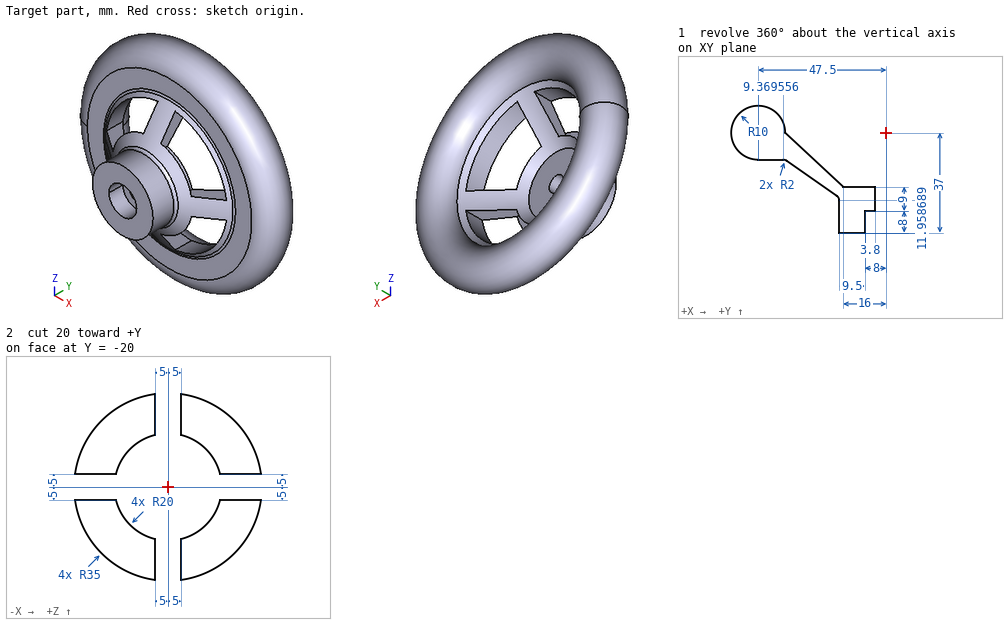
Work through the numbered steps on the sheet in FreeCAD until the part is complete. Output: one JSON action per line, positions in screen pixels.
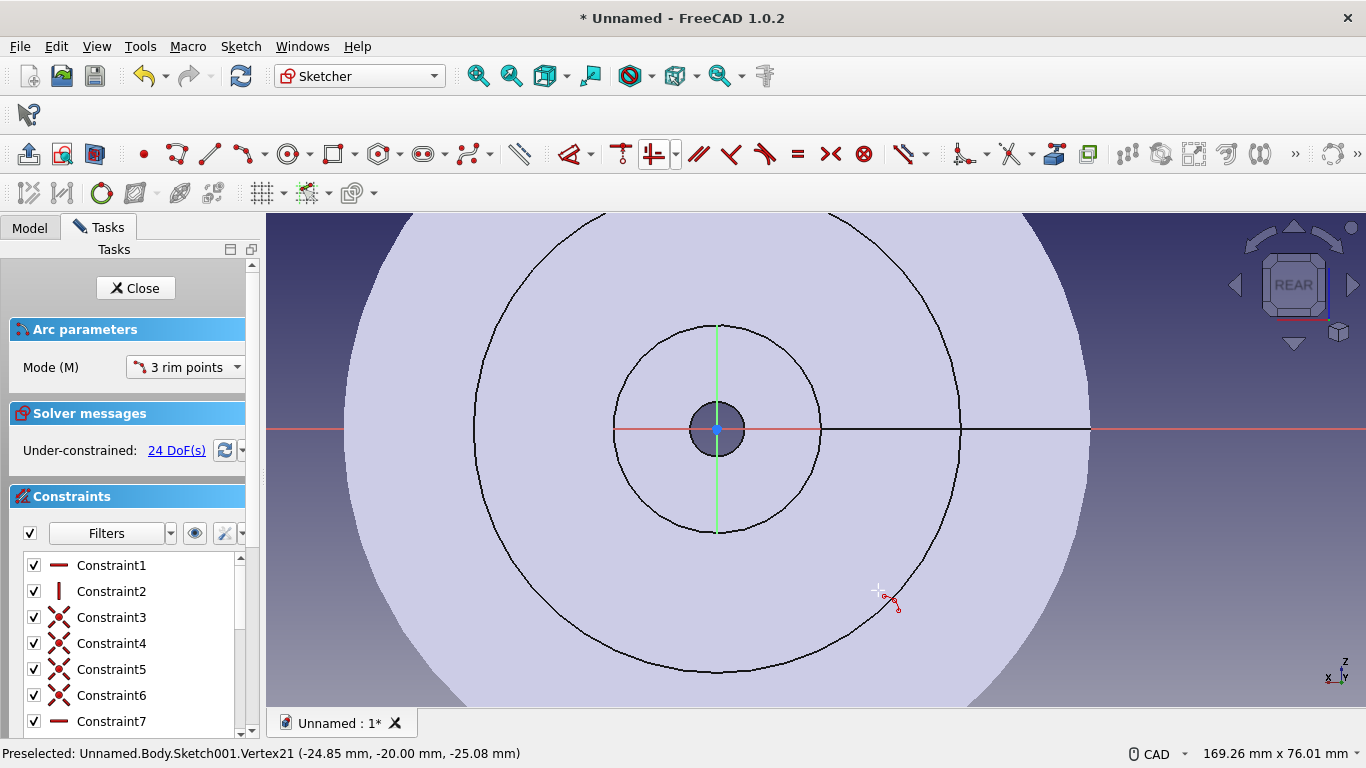
{"action": "key", "text": "g l"}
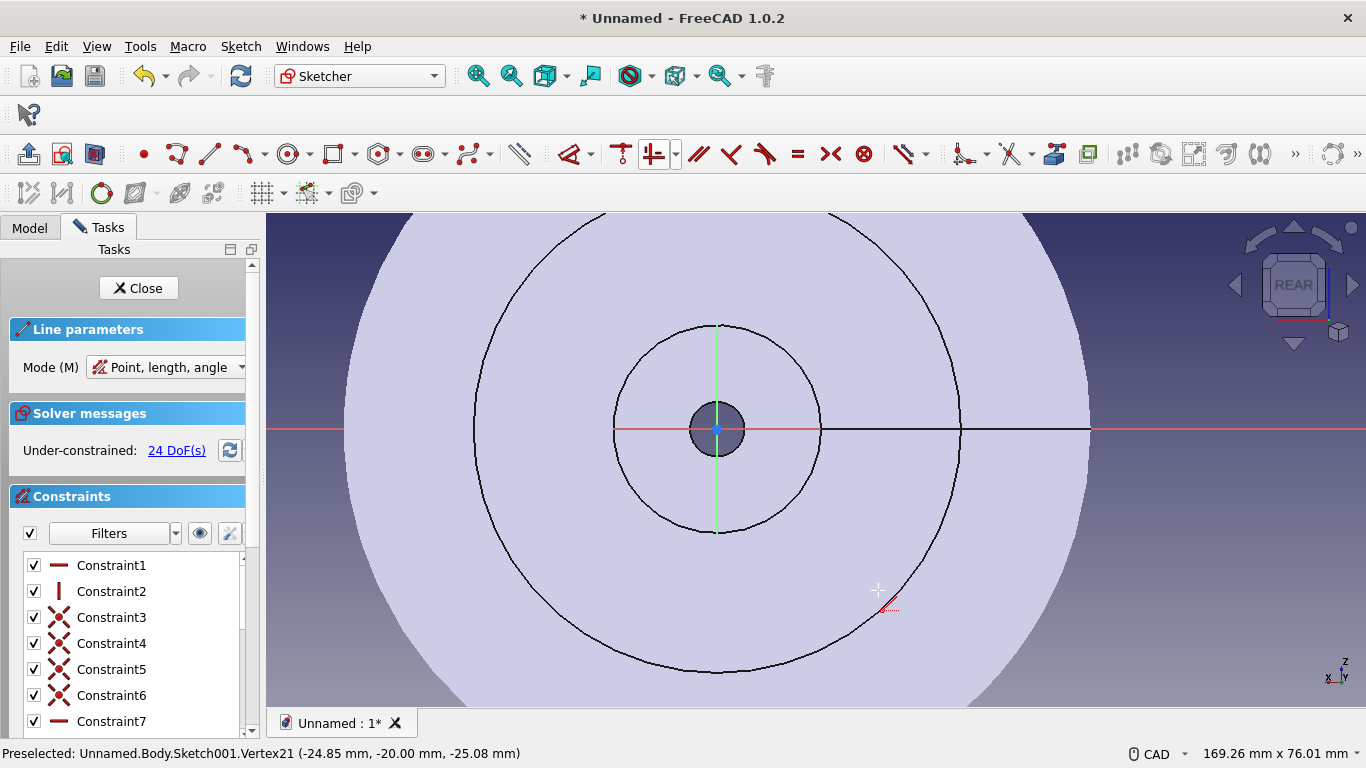
{"action": "scroll", "coordinate": [809, 523], "scroll_direction": "down", "scroll_amount": 2}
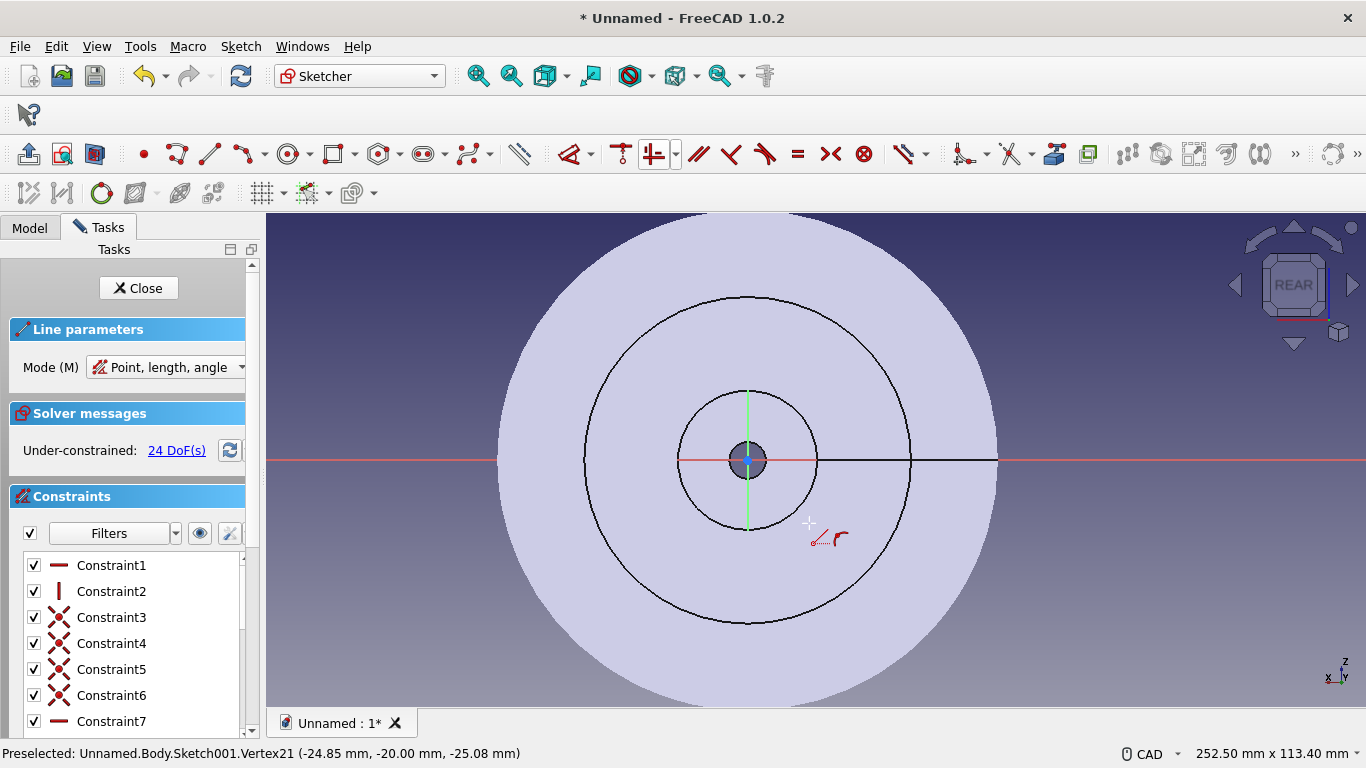
{"action": "left_click", "coordinate": [769, 309]}
{"action": "left_click", "coordinate": [769, 376]}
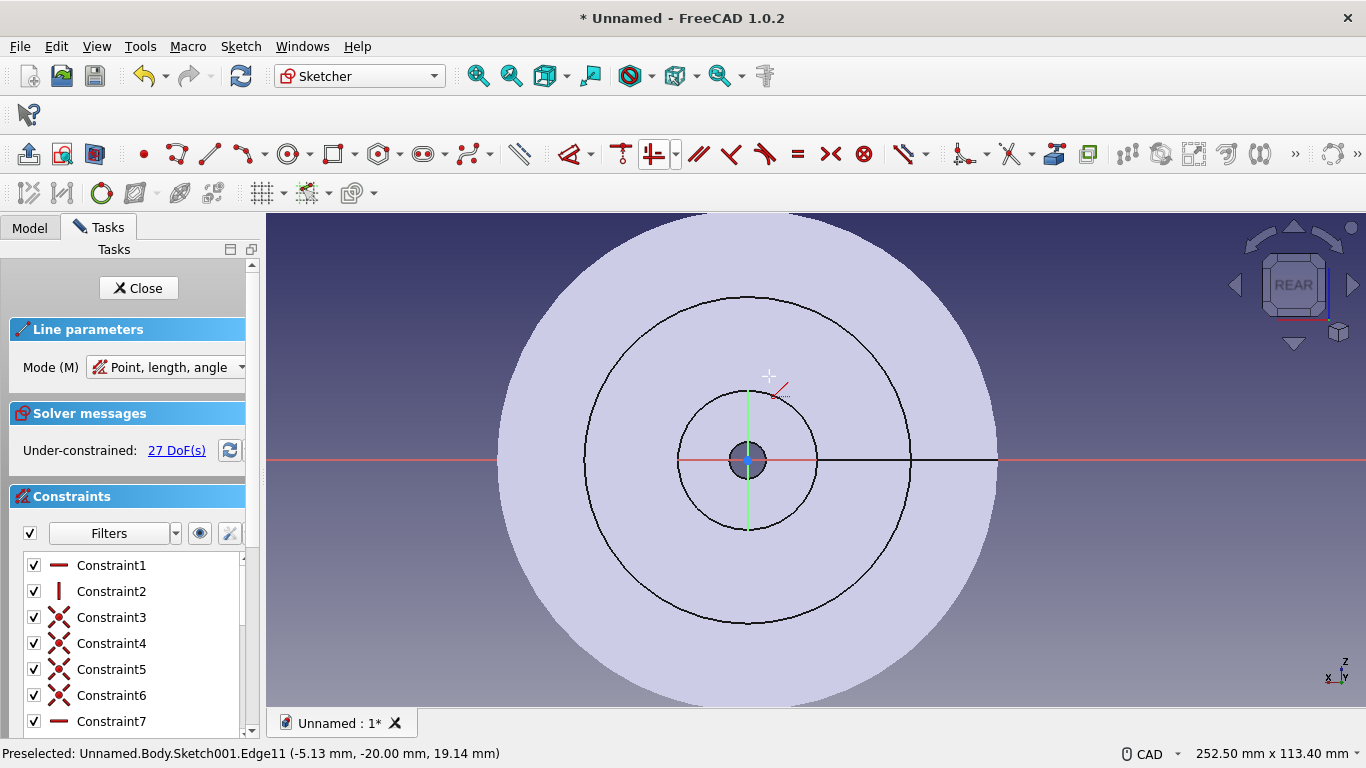
{"action": "left_click", "coordinate": [832, 439]}
{"action": "left_click", "coordinate": [899, 439]}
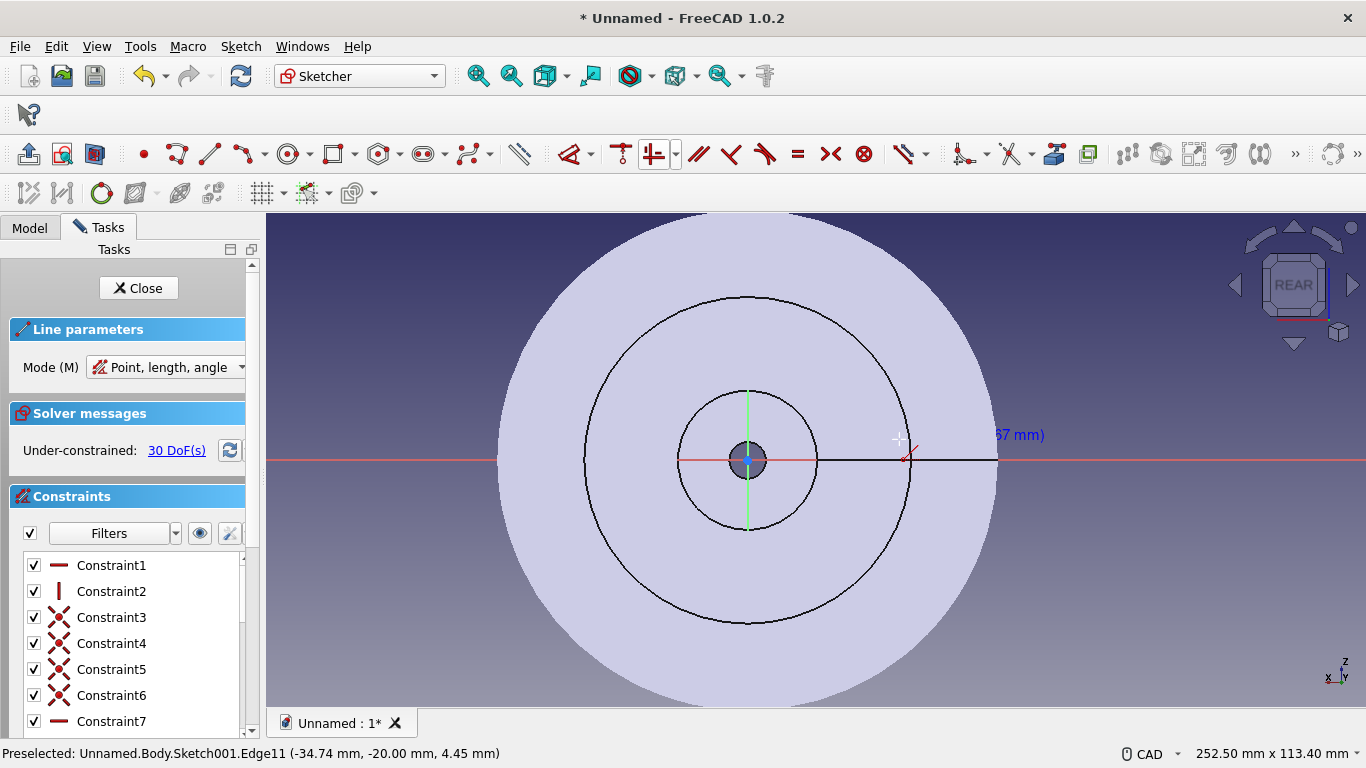
{"action": "left_click", "coordinate": [242, 154]}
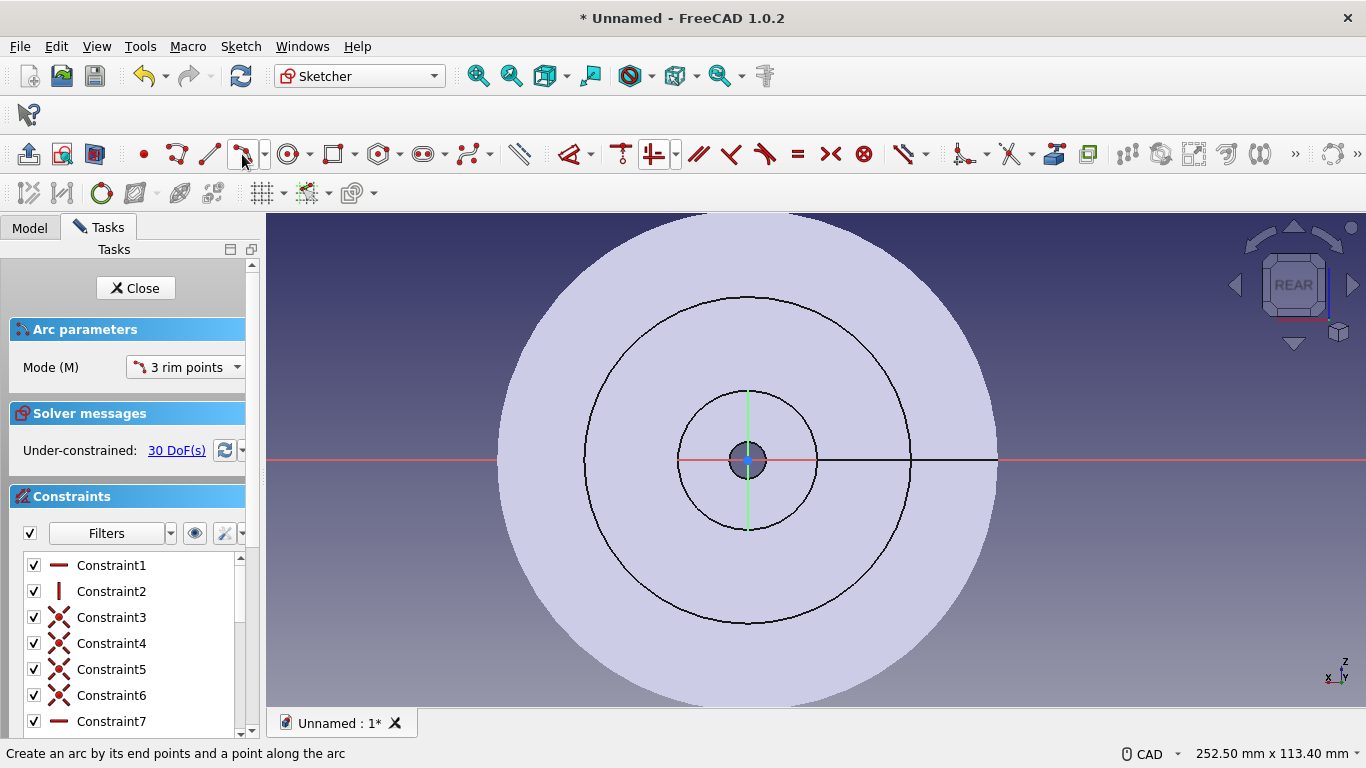
{"action": "left_click", "coordinate": [769, 377]}
{"action": "left_click", "coordinate": [832, 440]}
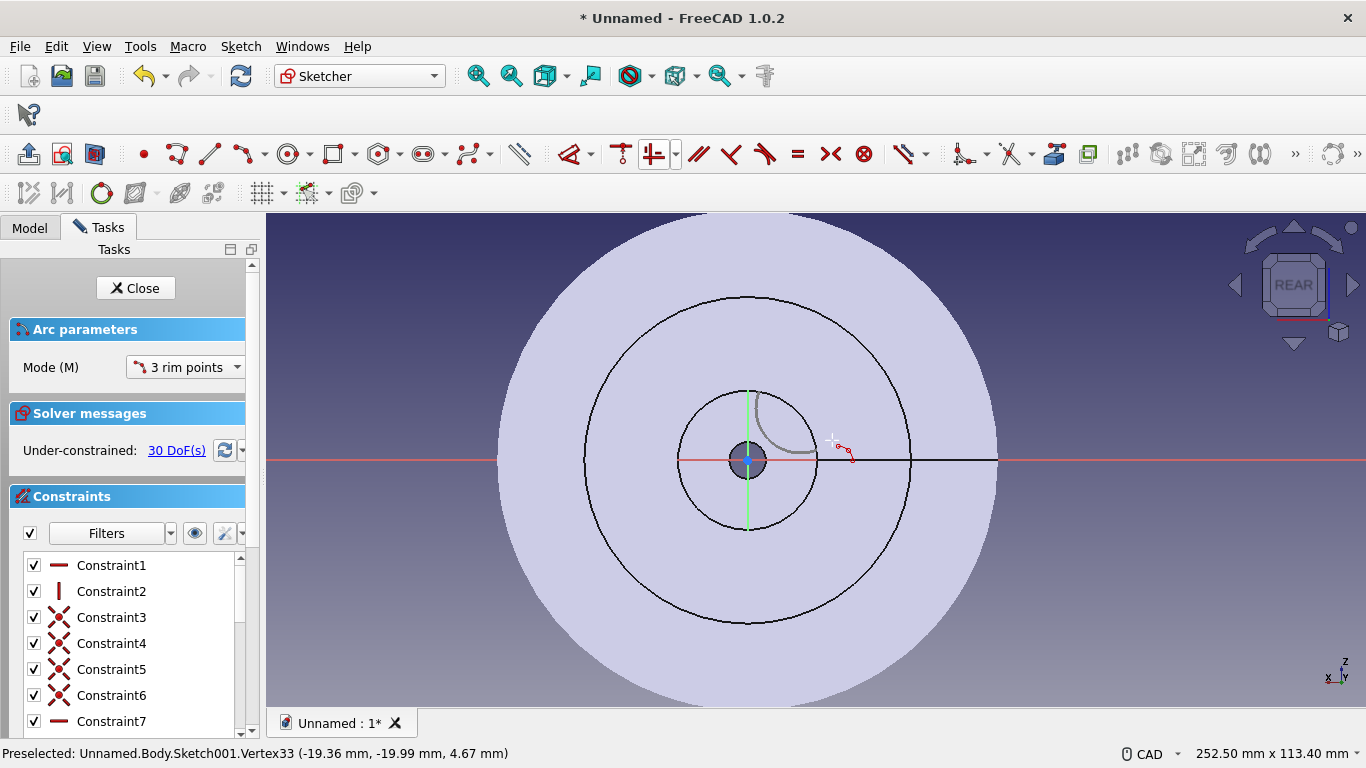
{"action": "scroll", "coordinate": [809, 399], "scroll_direction": "up", "scroll_amount": 2}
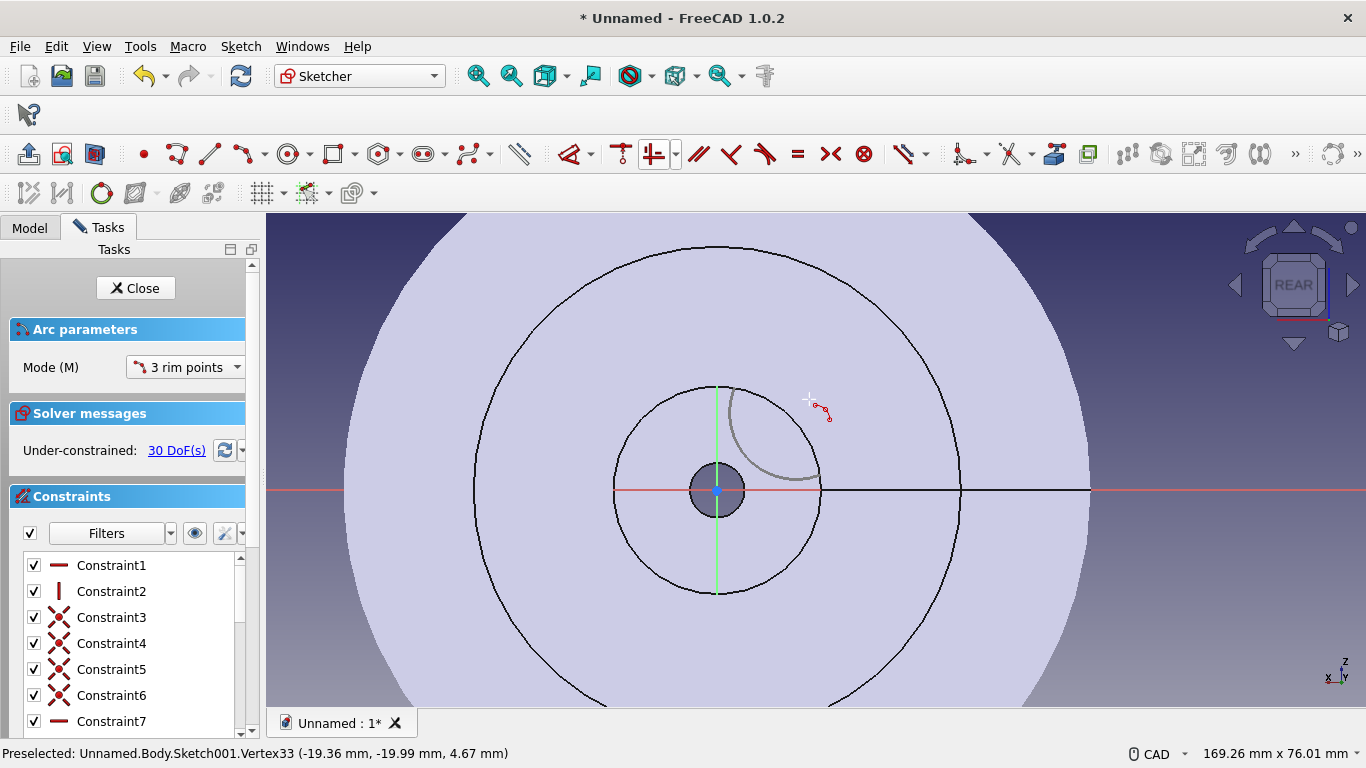
{"action": "left_click", "coordinate": [809, 398]}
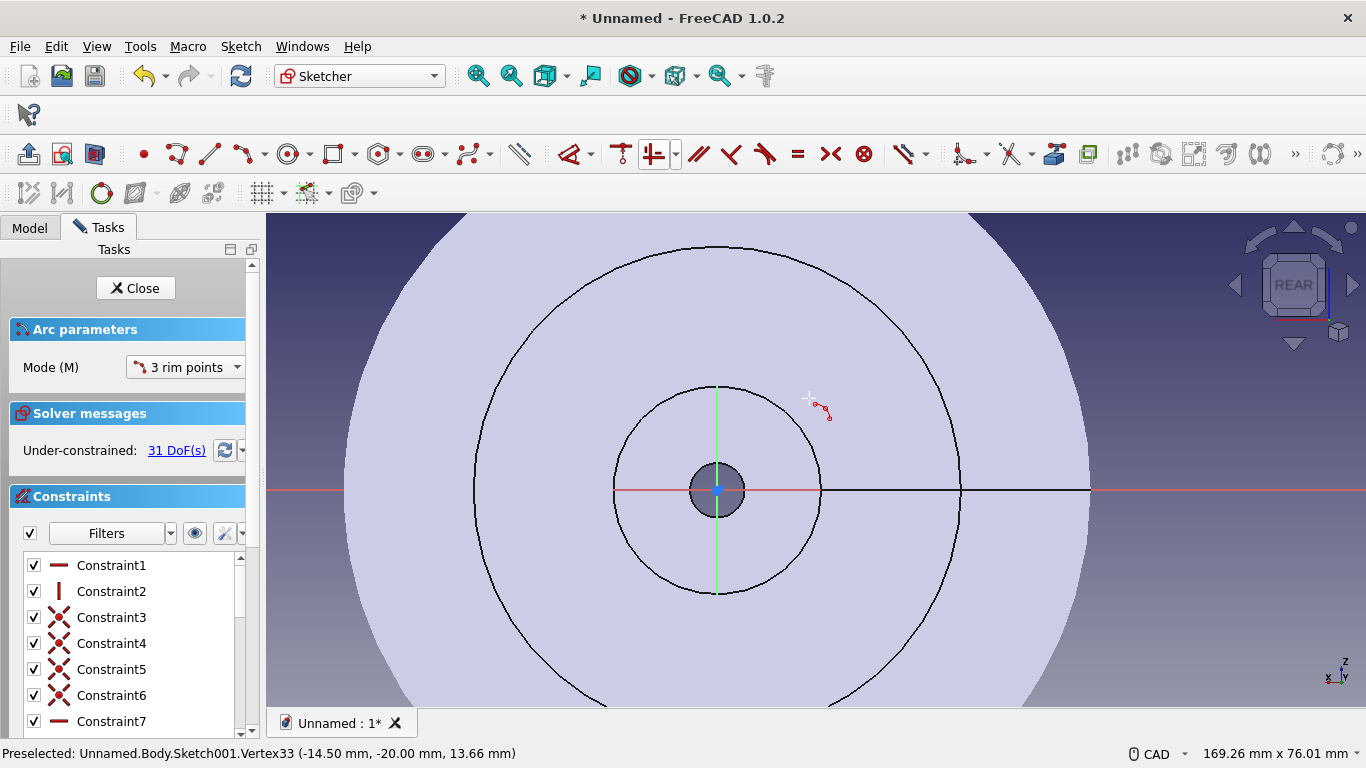
{"action": "left_click", "coordinate": [943, 460]}
{"action": "left_click", "coordinate": [749, 266]}
{"action": "left_click", "coordinate": [878, 329]}
{"action": "key", "text": "Escape"}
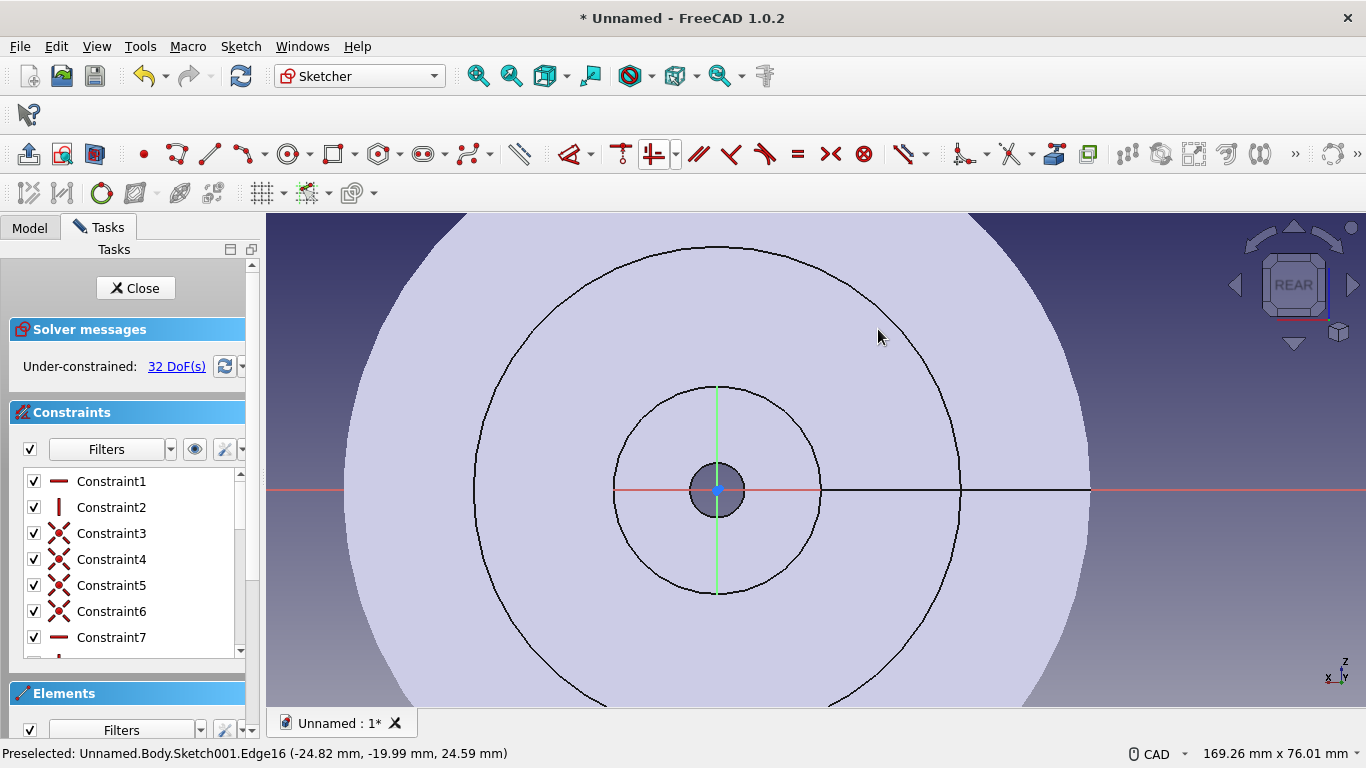
{"action": "left_click", "coordinate": [521, 606]}